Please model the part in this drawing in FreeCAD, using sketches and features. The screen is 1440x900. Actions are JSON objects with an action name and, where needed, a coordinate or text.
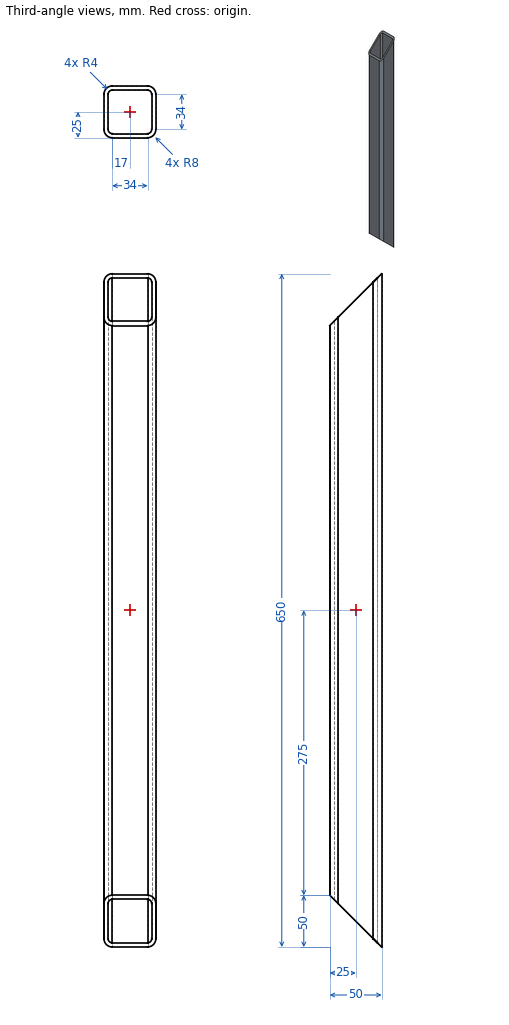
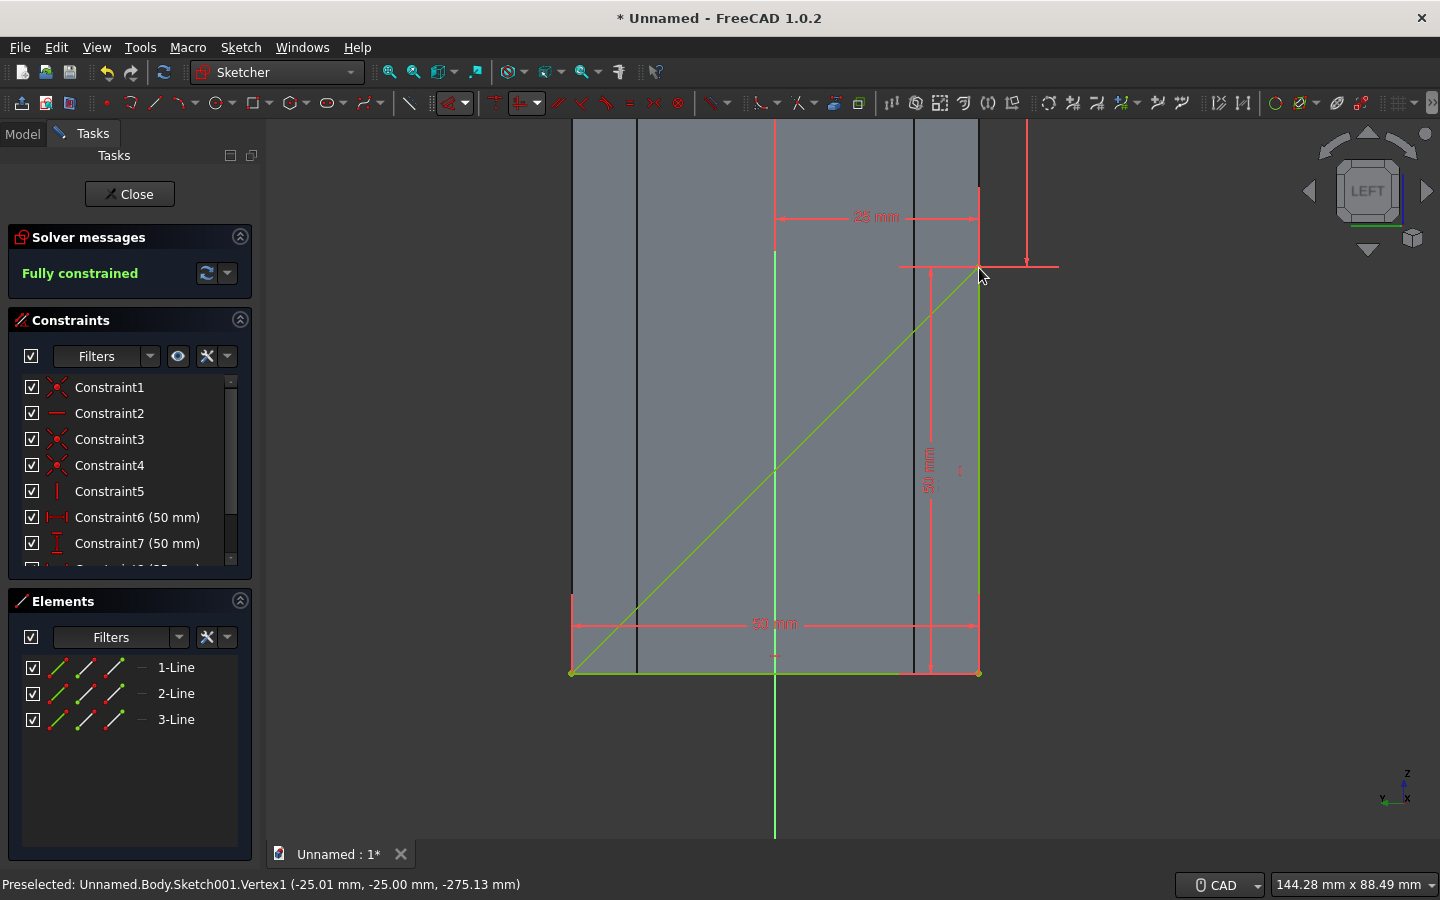
{"action": "left_click", "coordinate": [130, 194]}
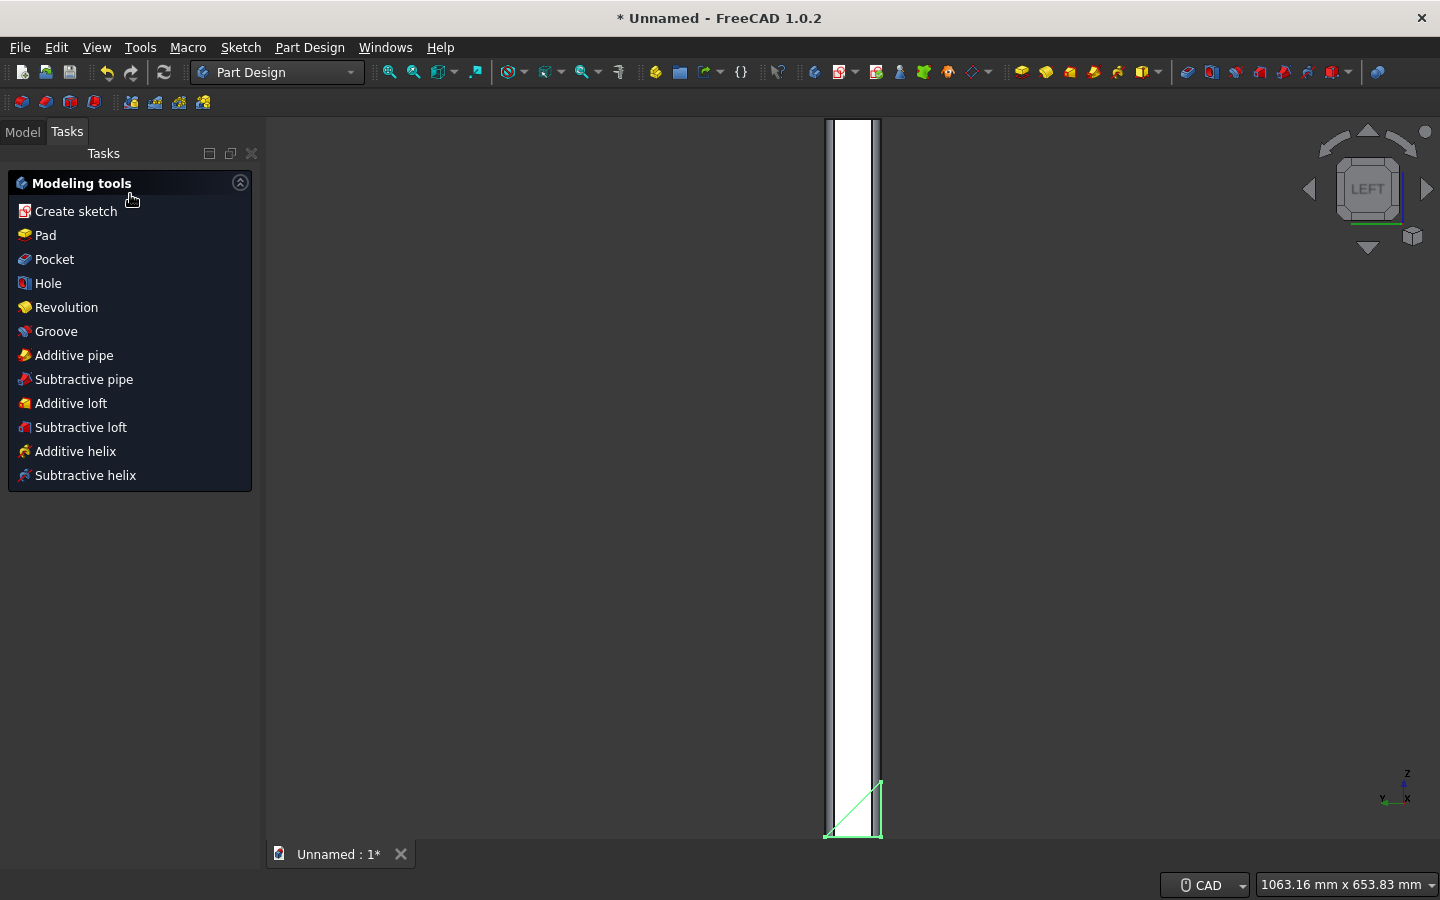
{"action": "left_click", "coordinate": [1188, 72]}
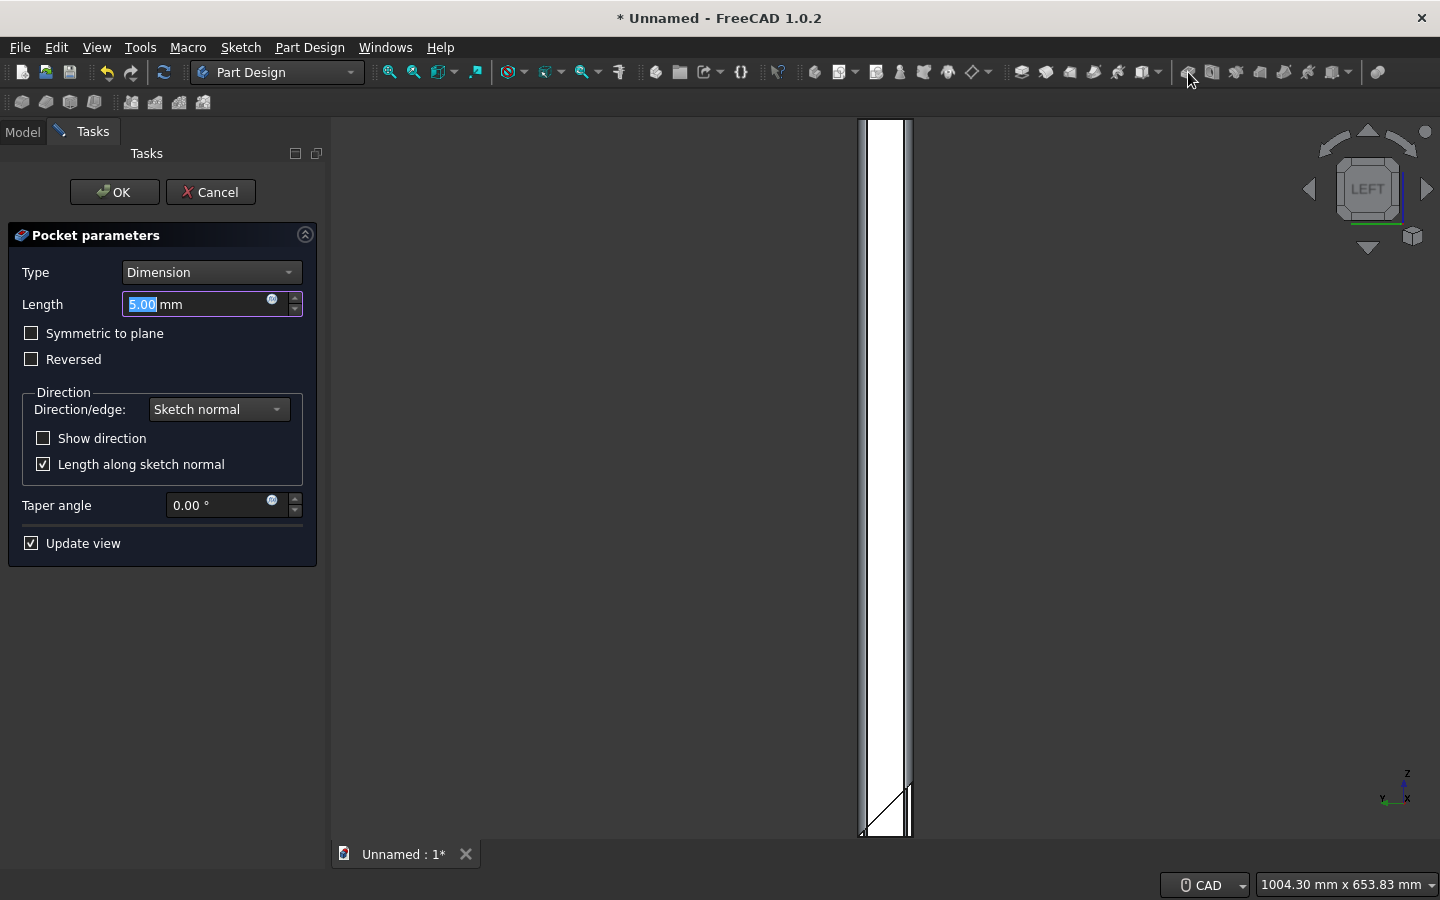
{"action": "left_click", "coordinate": [212, 272]}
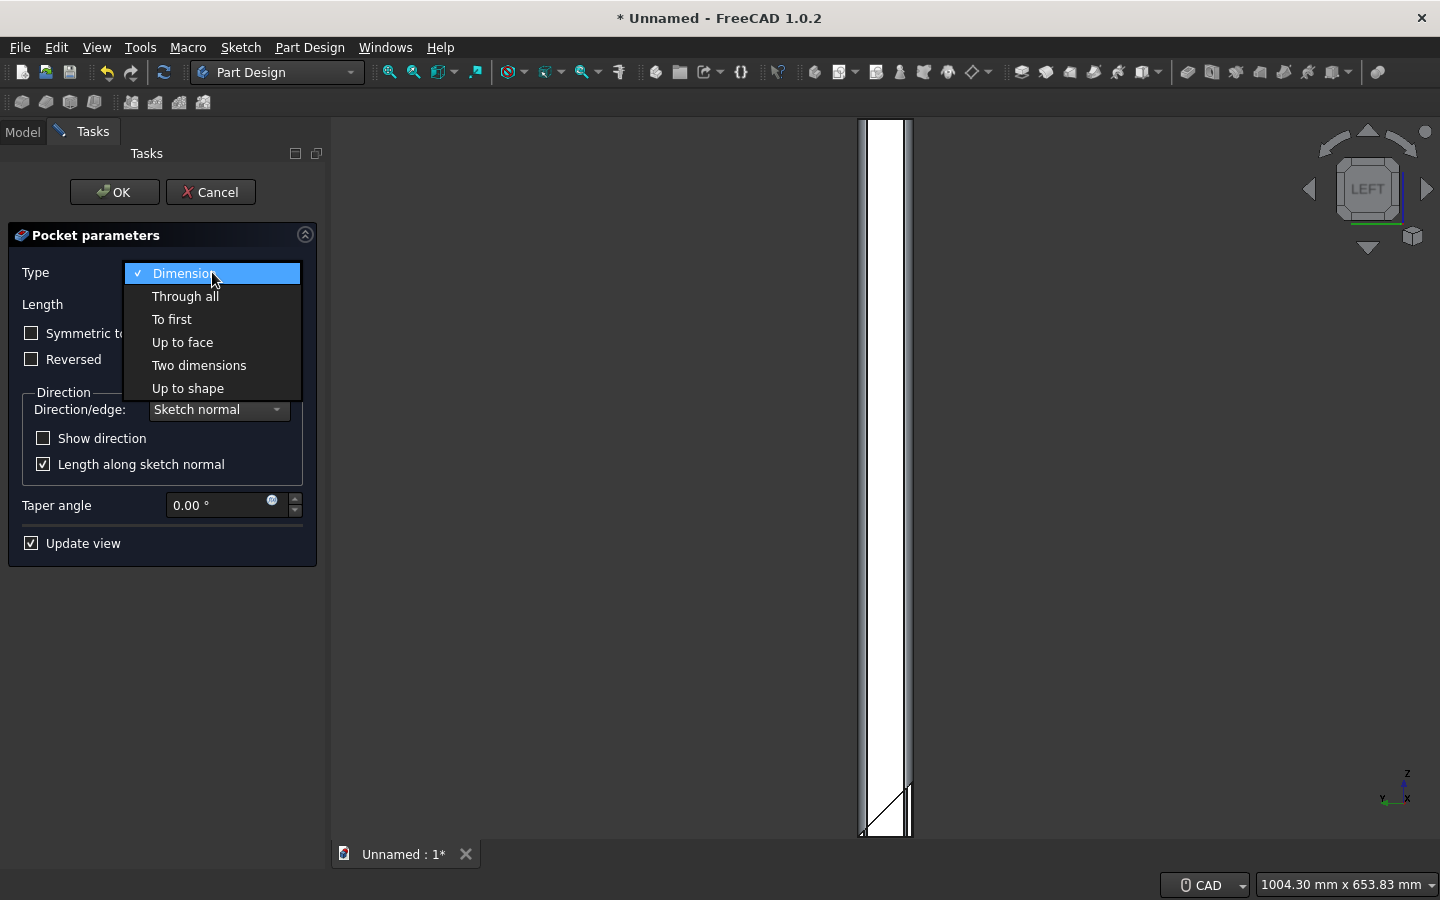
{"action": "left_click", "coordinate": [212, 296]}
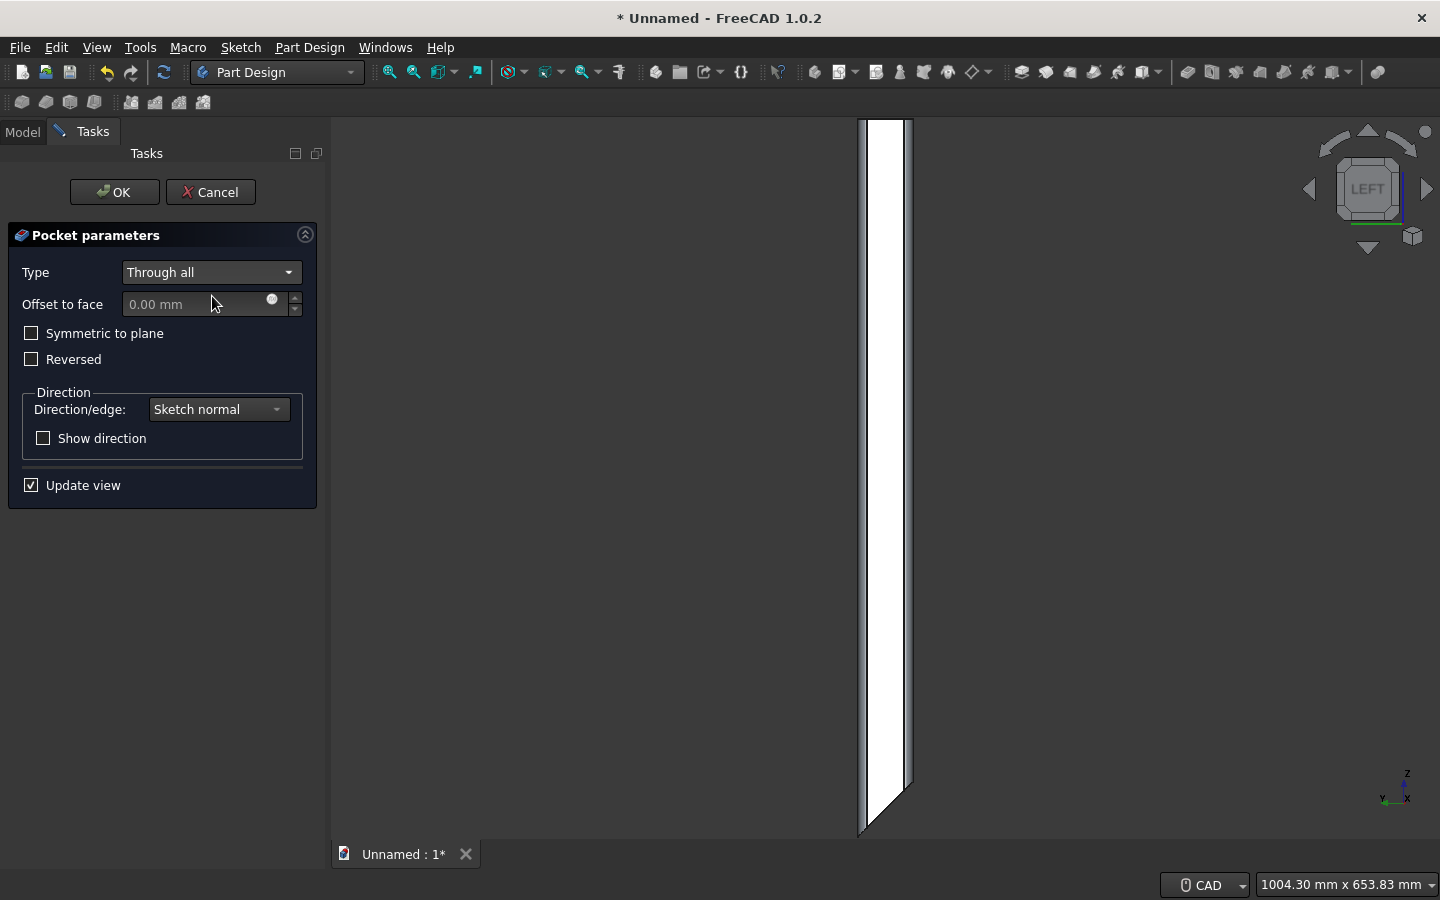
{"action": "left_click", "coordinate": [115, 192]}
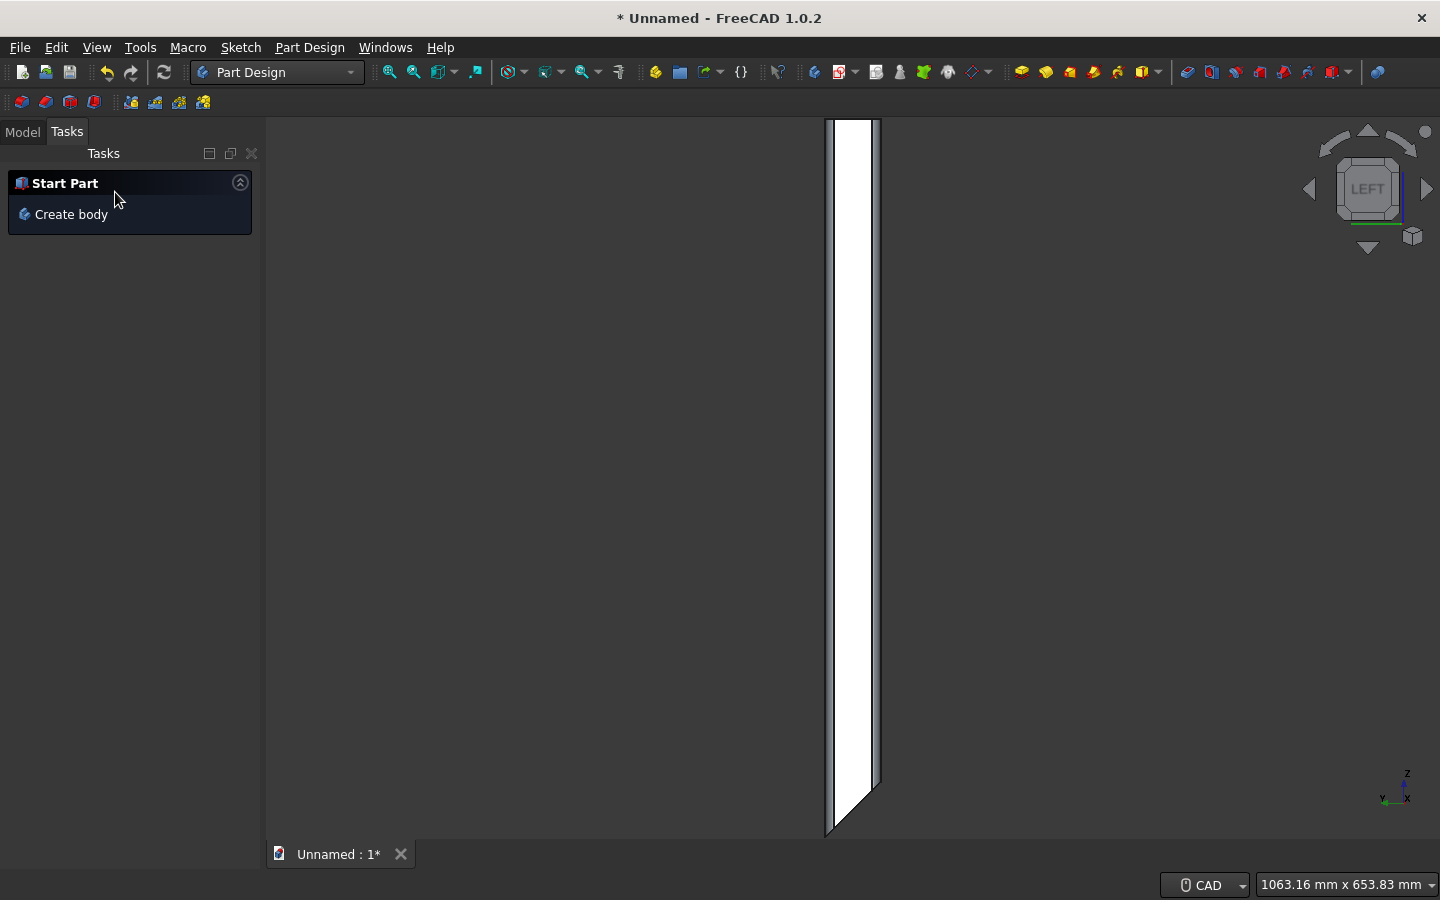
{"action": "left_click", "coordinate": [23, 131]}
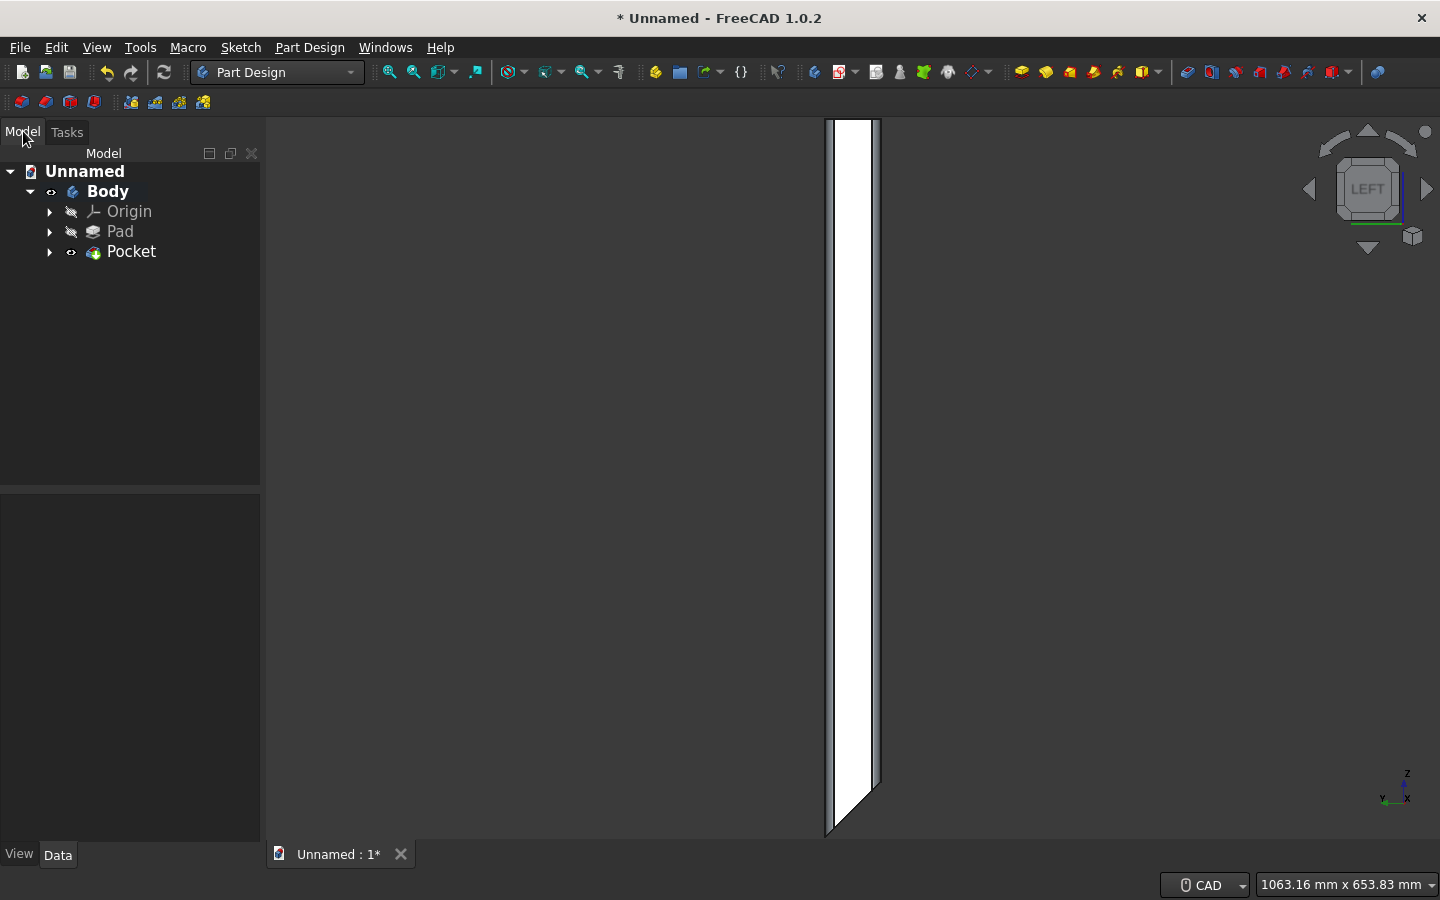
{"action": "left_click", "coordinate": [116, 252]}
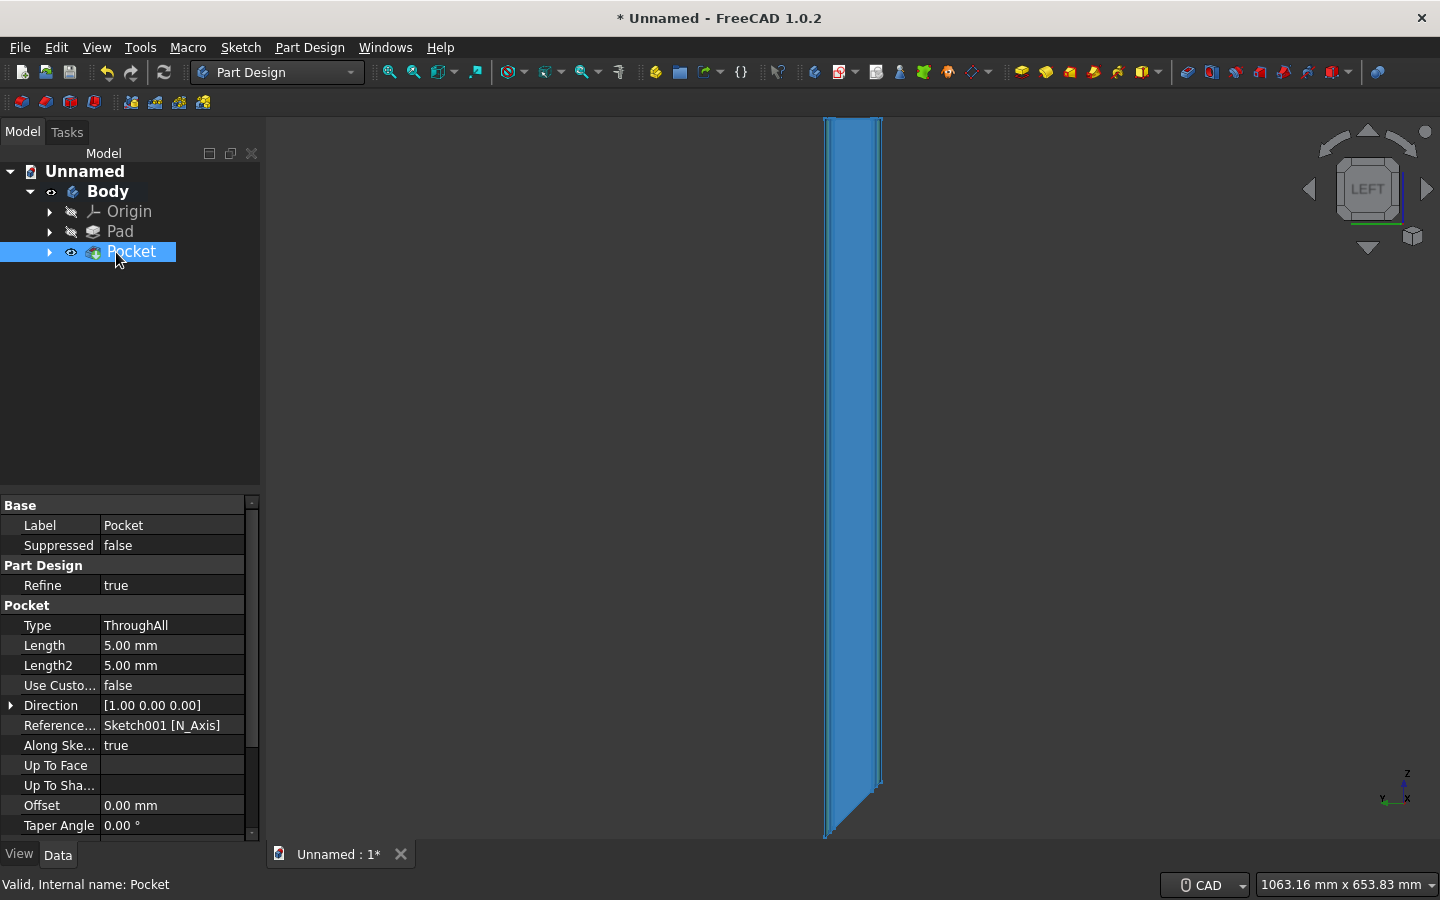
{"action": "left_click", "coordinate": [132, 102]}